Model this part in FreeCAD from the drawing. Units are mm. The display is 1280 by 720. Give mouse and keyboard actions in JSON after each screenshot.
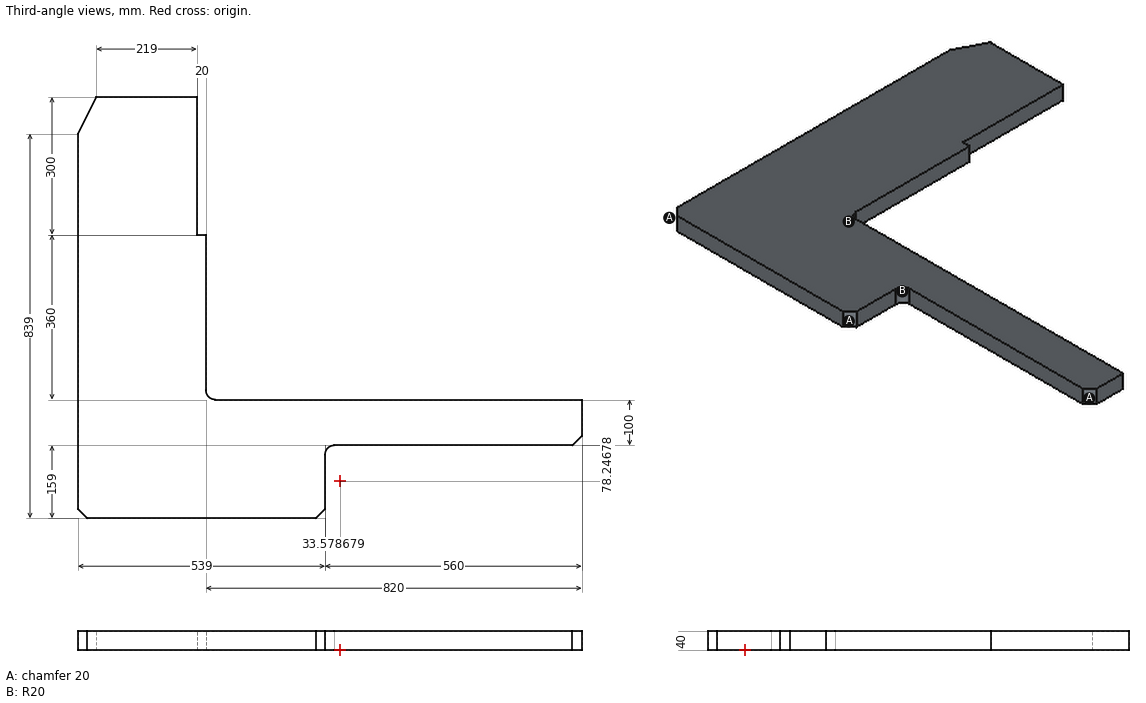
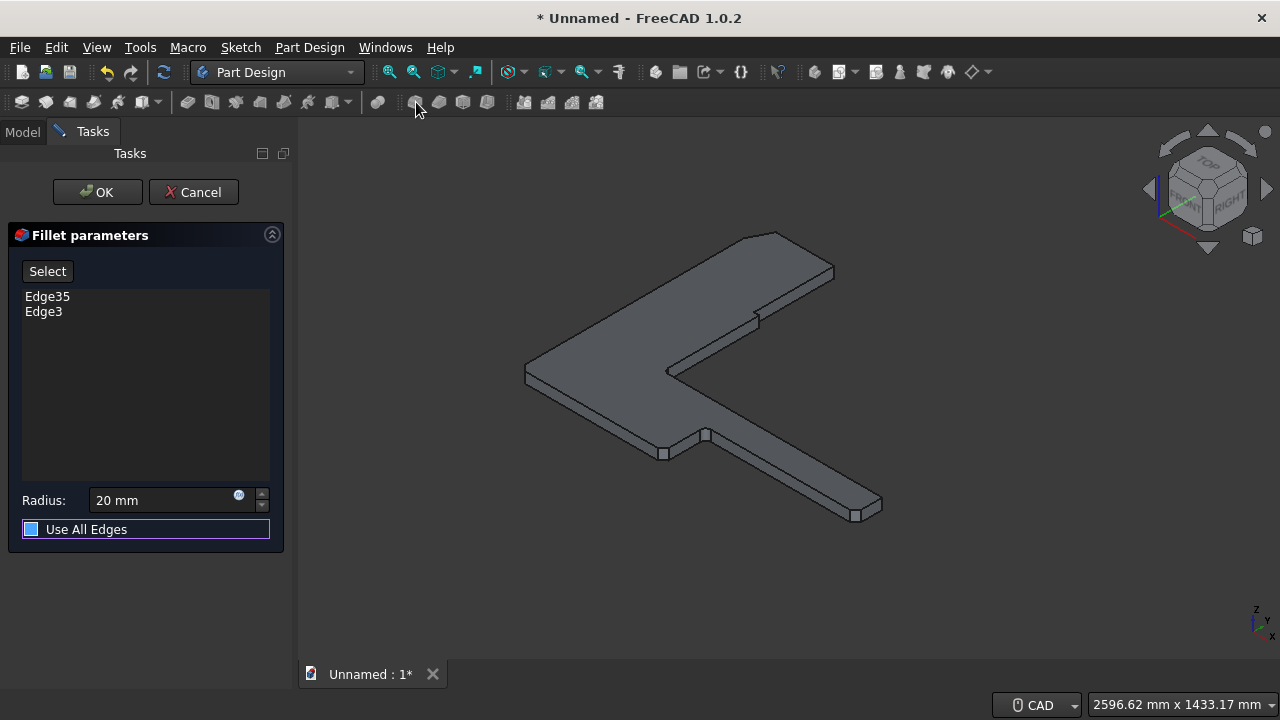
{"action": "left_click", "coordinate": [98, 192]}